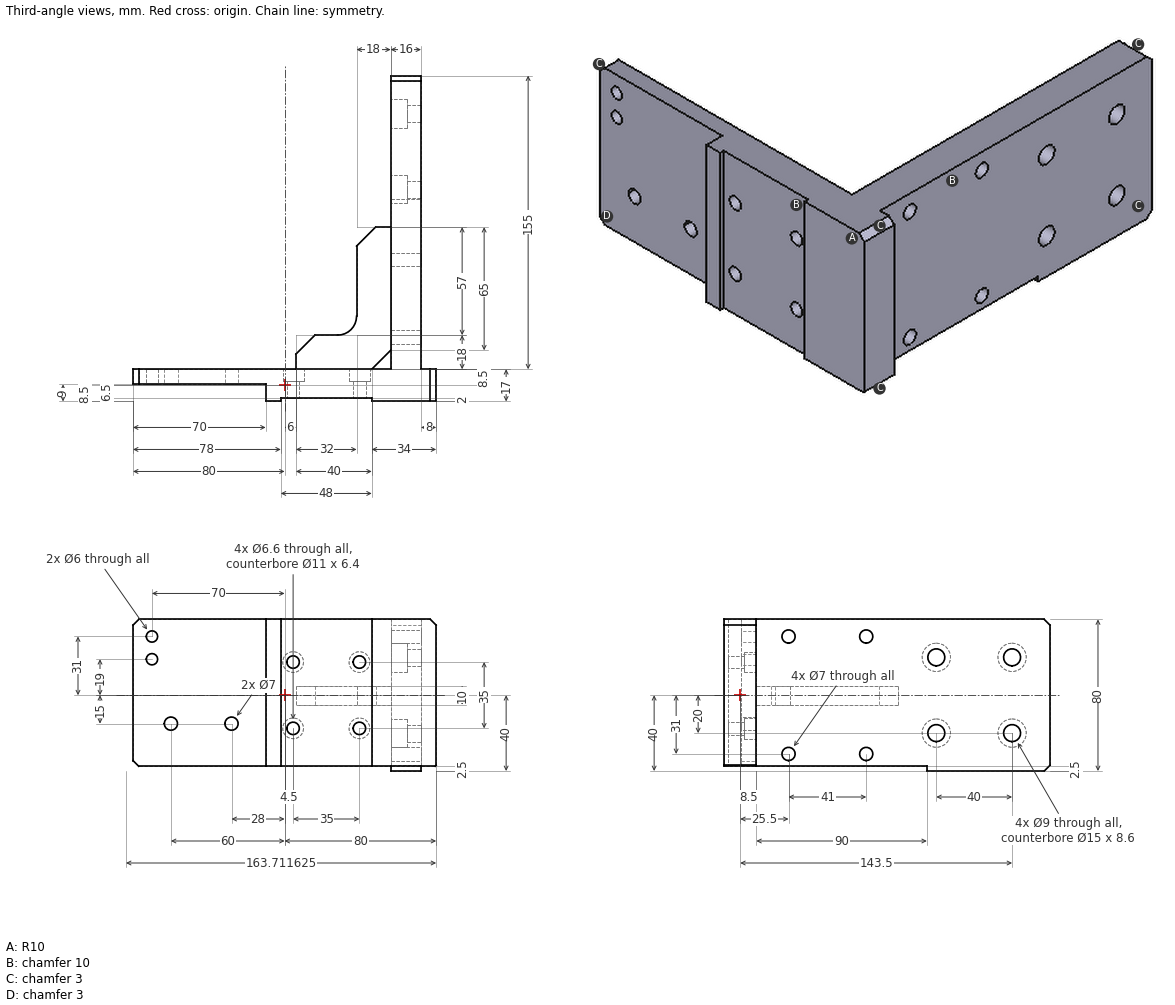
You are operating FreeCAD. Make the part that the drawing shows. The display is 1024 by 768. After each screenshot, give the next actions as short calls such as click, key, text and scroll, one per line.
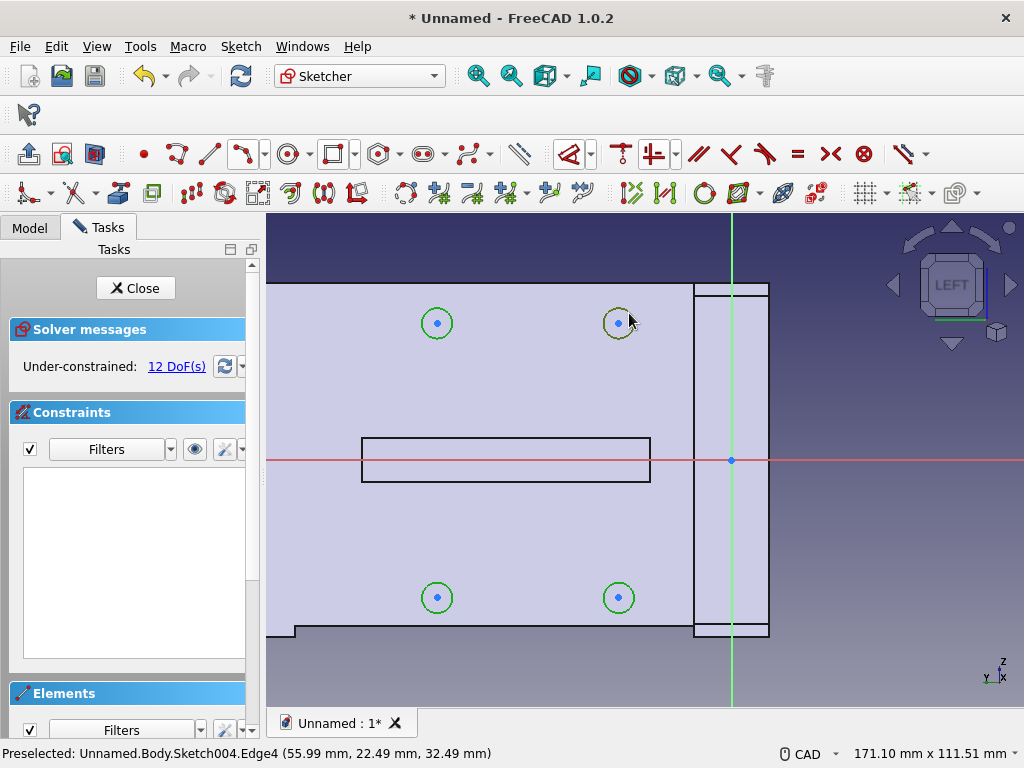
click(798, 154)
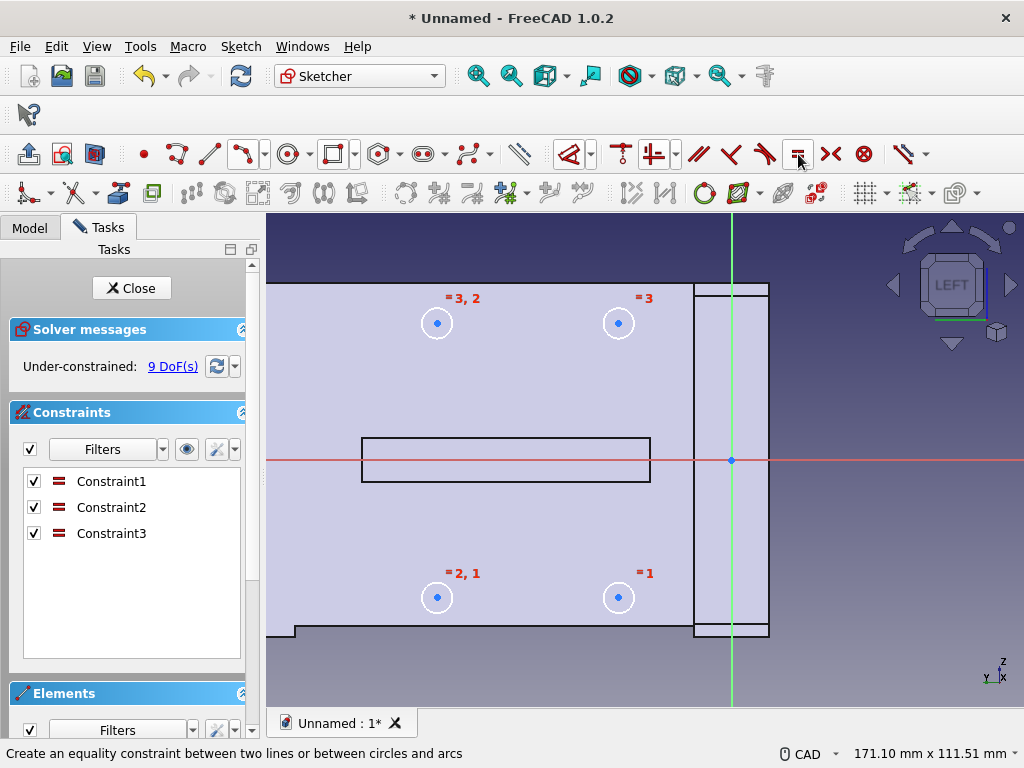
click(437, 598)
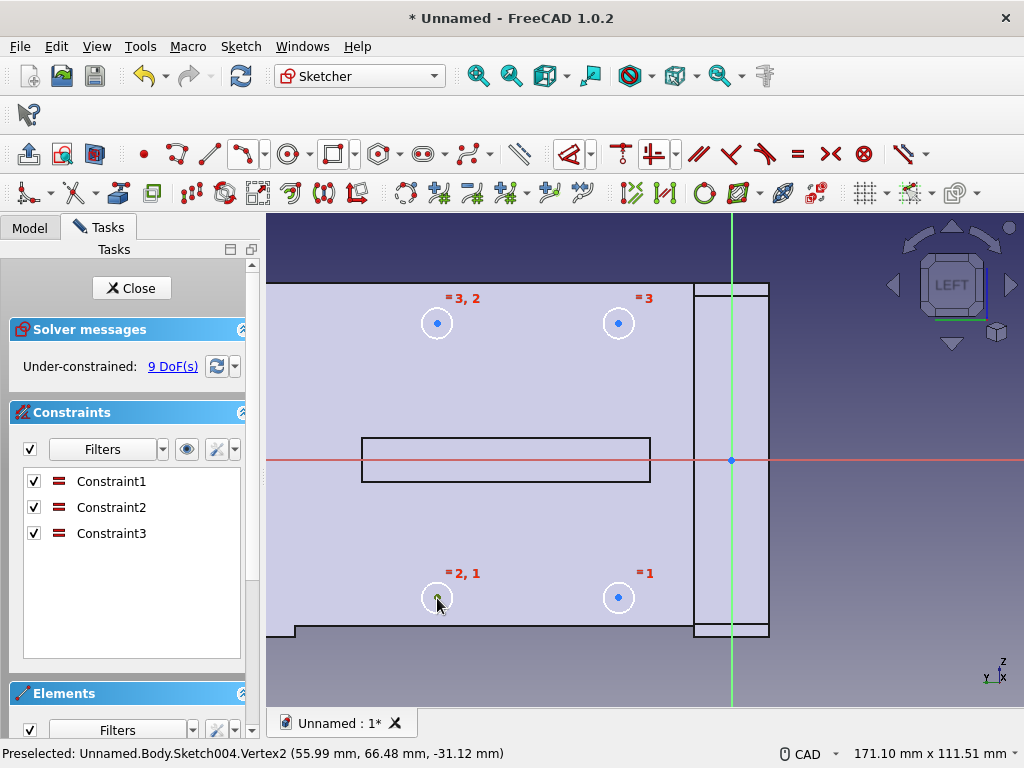
click(437, 323)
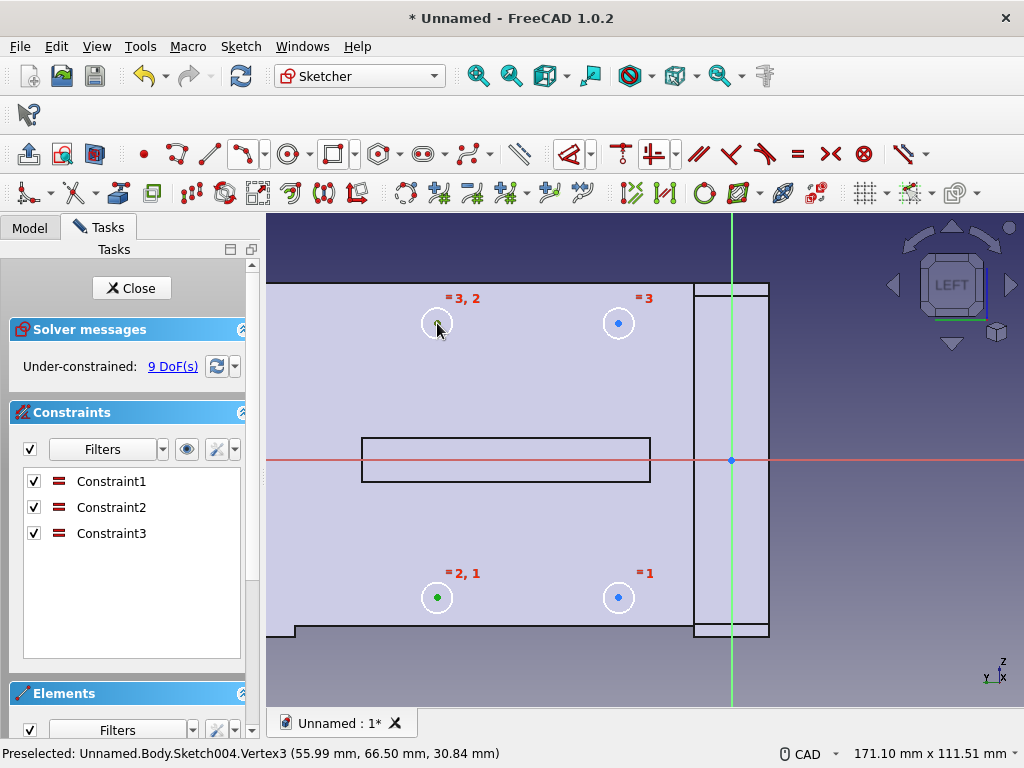
click(334, 460)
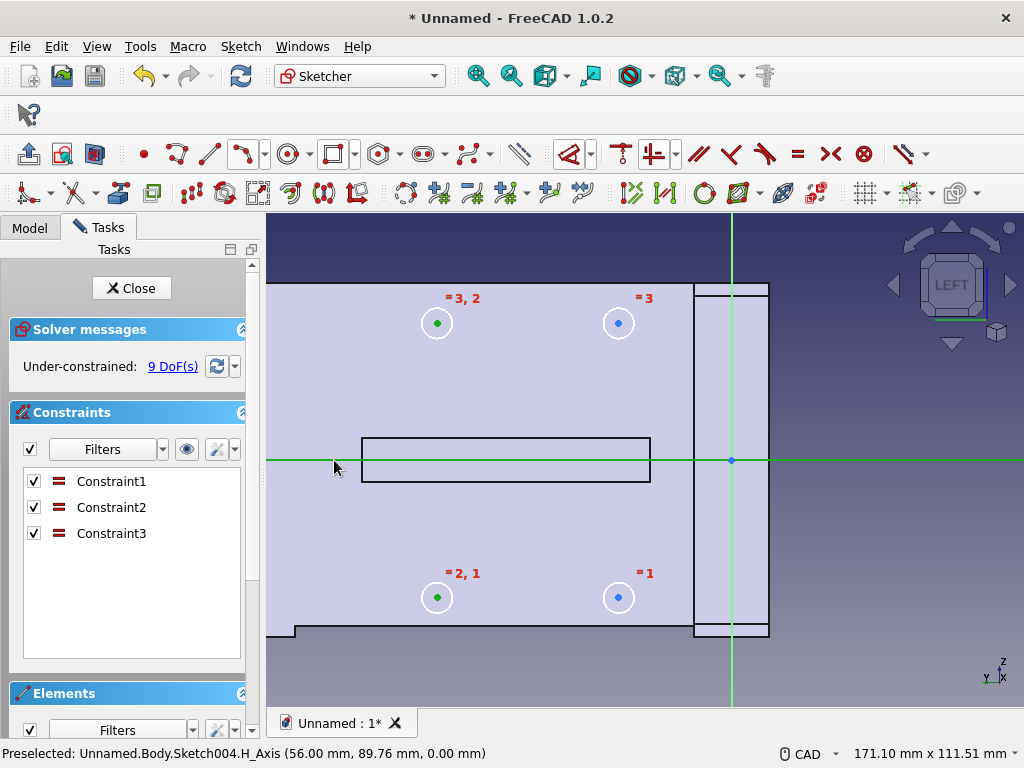
click(831, 154)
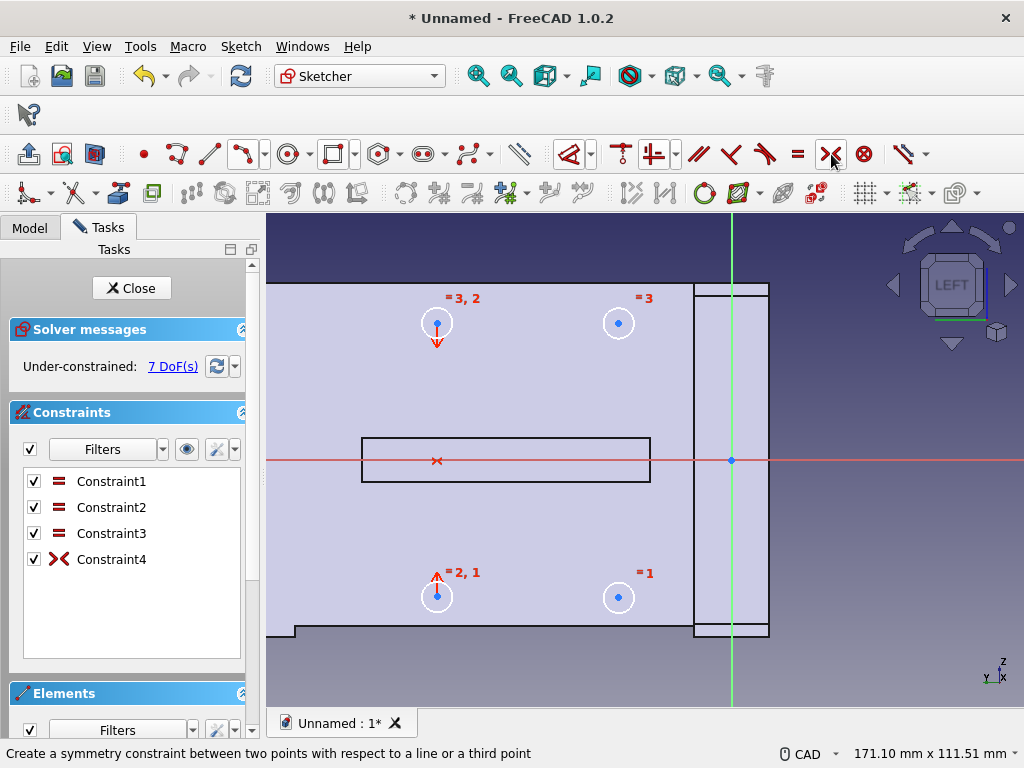
click(619, 598)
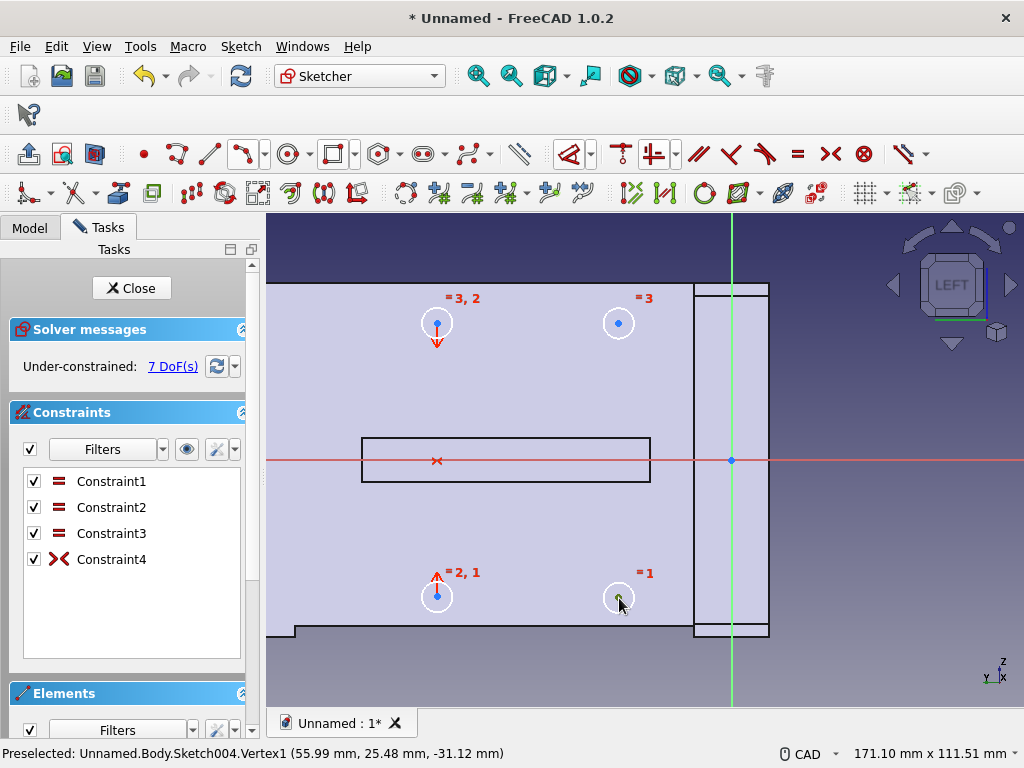
click(619, 323)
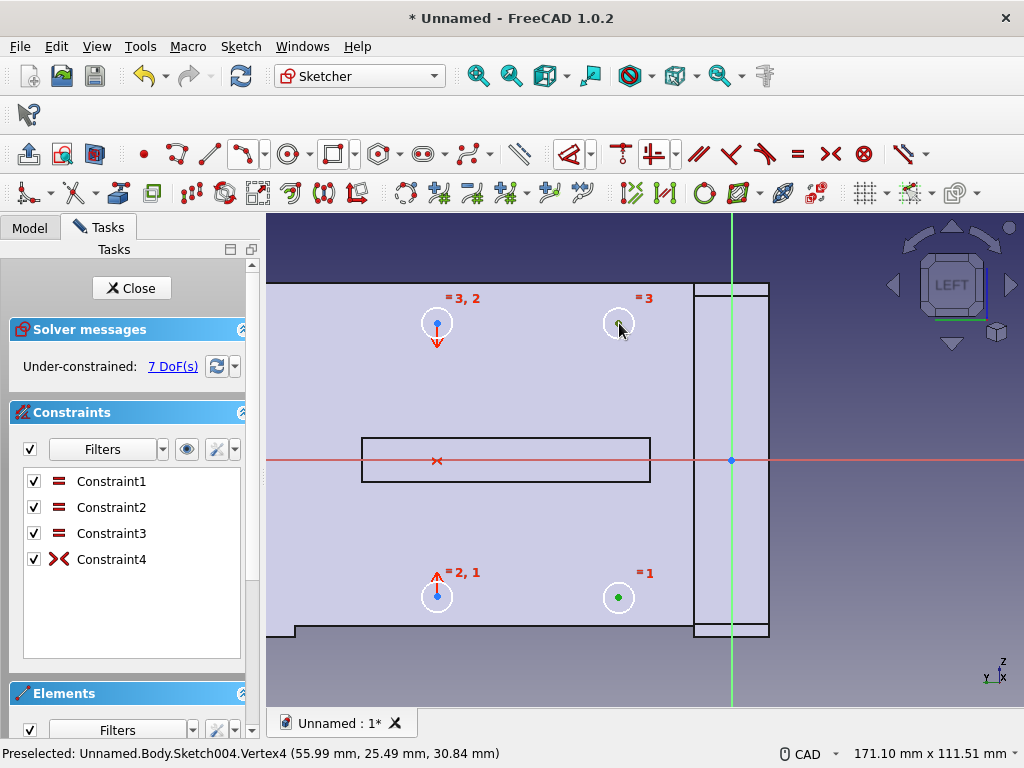
click(334, 460)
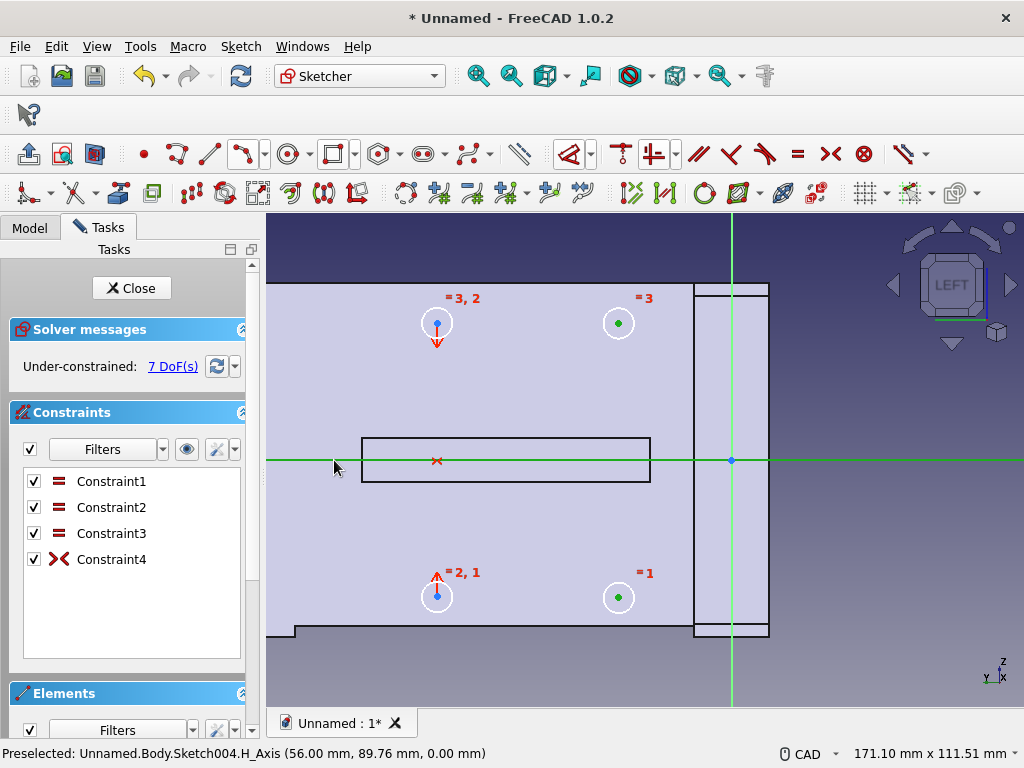
click(831, 154)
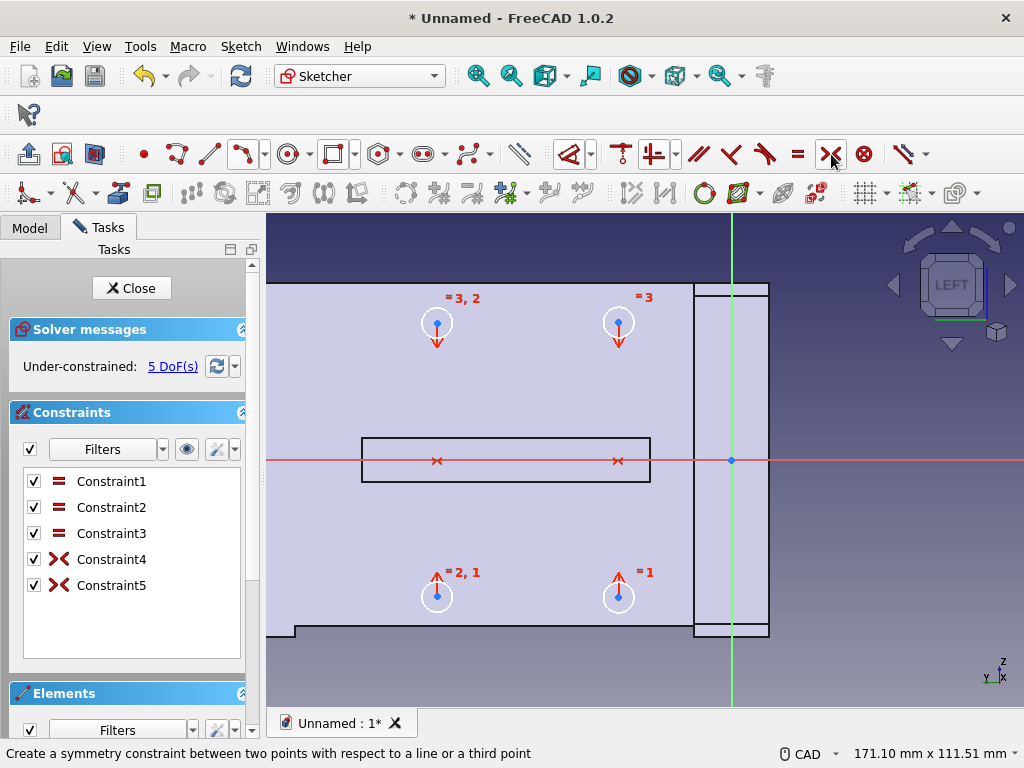
scroll(629, 587, up, 2)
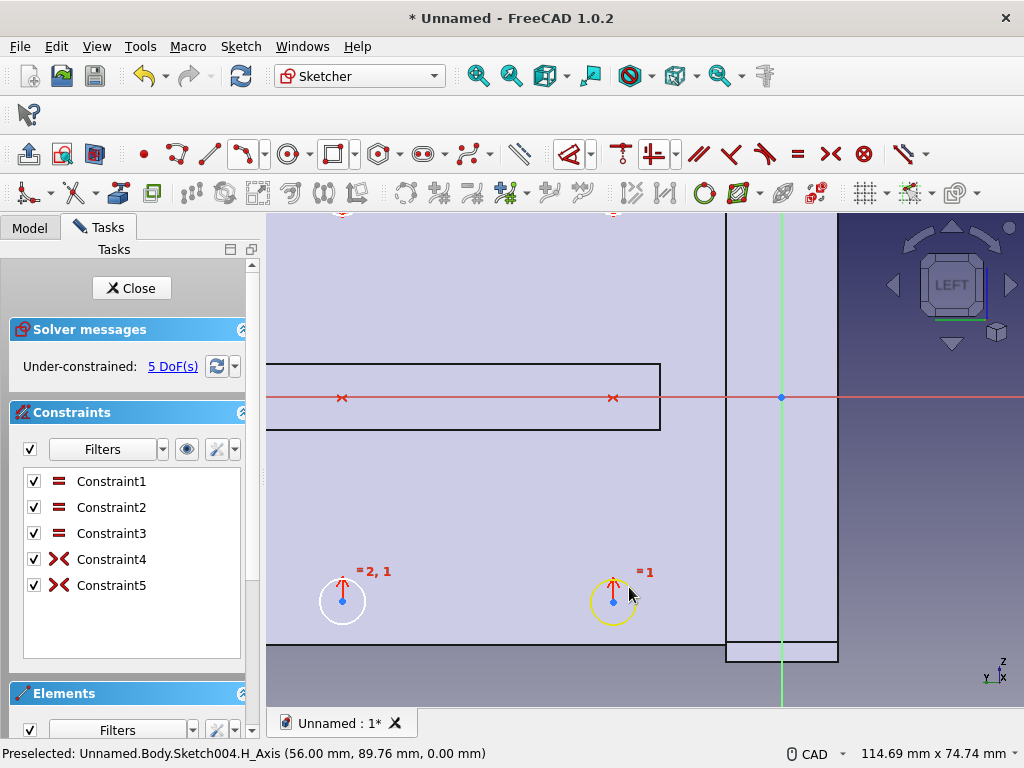
click(629, 586)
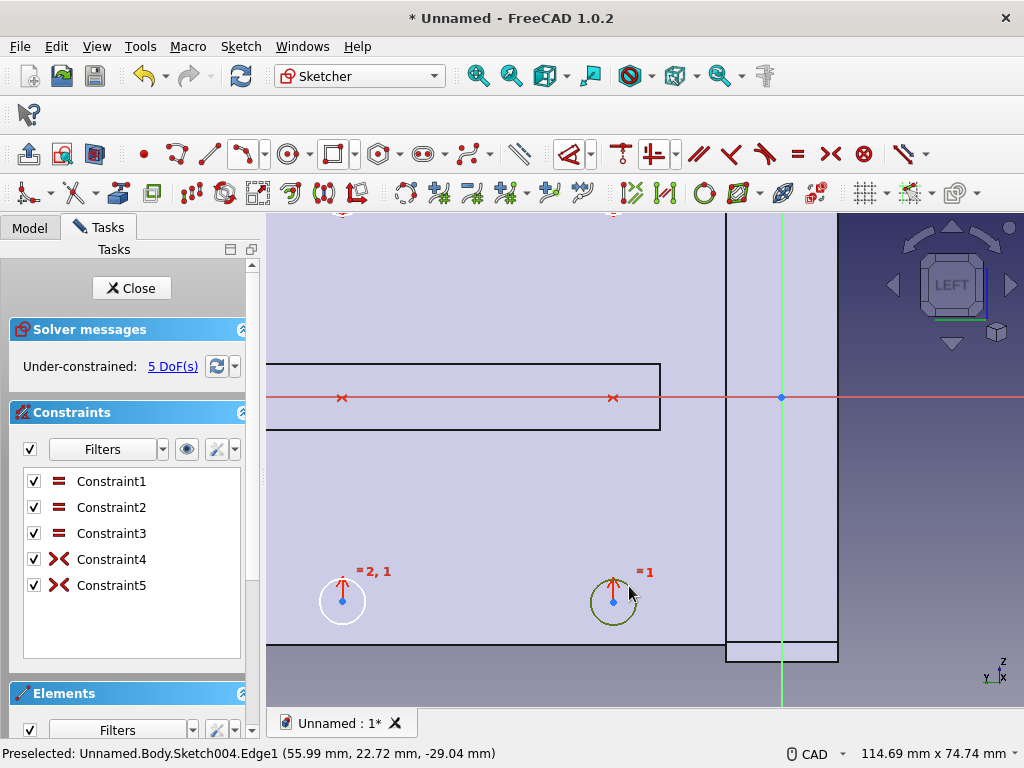
key(k)
key(o)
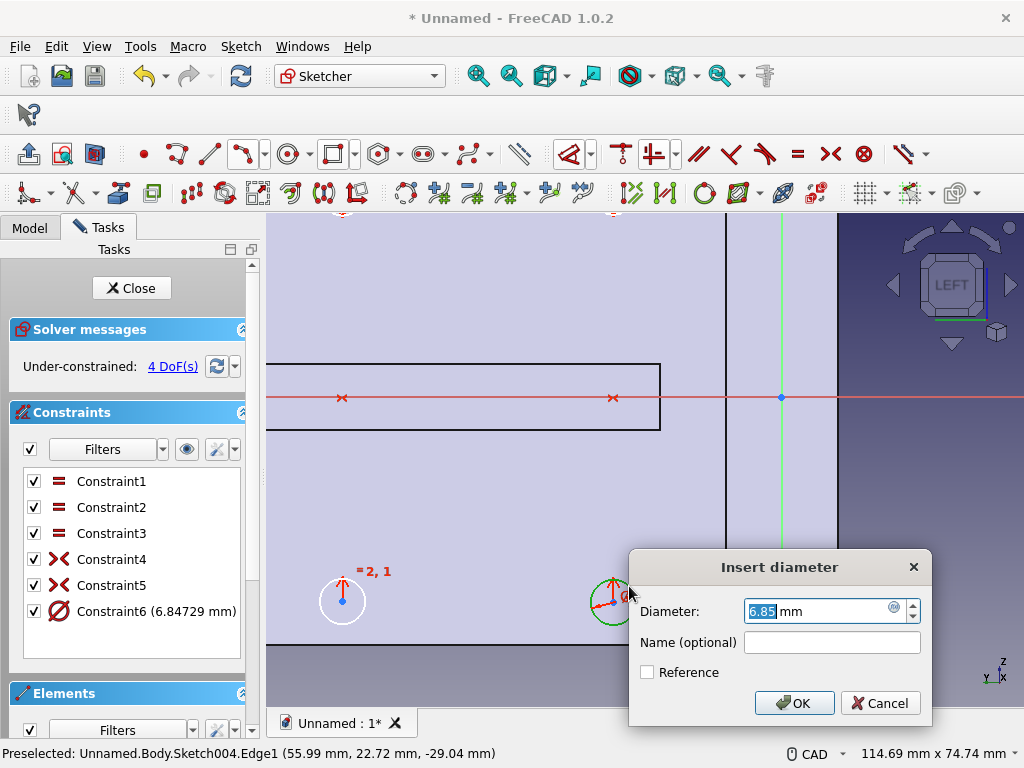
text(7)
key(Return)